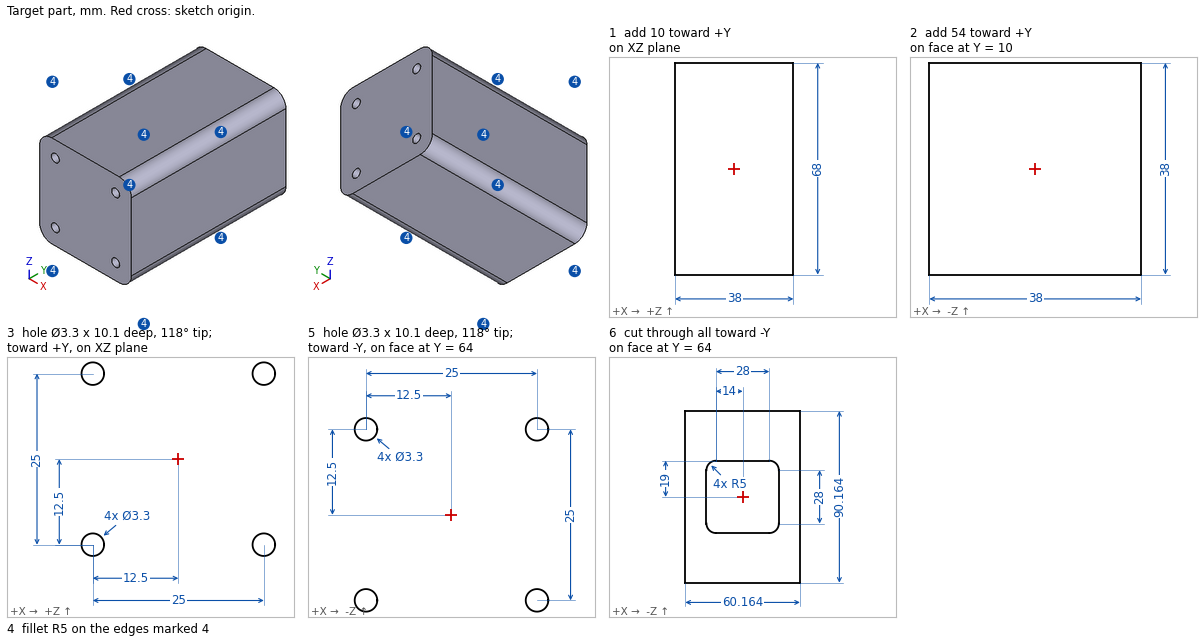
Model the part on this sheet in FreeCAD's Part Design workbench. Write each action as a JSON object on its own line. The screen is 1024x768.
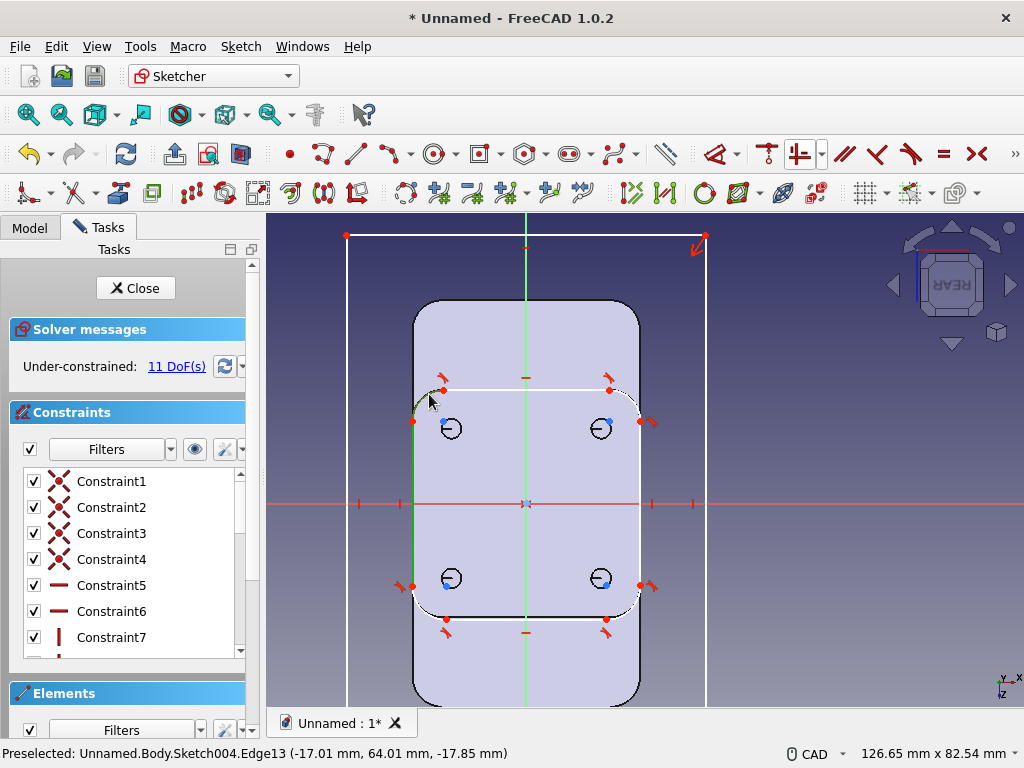
{"action": "left_click", "coordinate": [911, 154]}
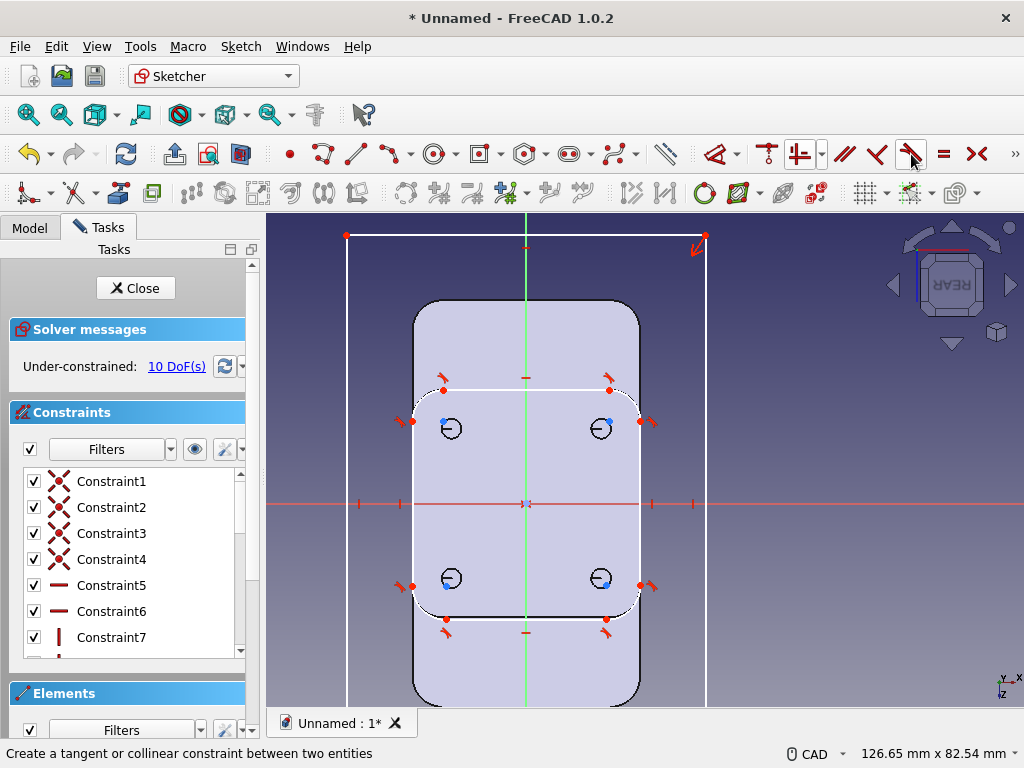
{"action": "left_click", "coordinate": [637, 407]}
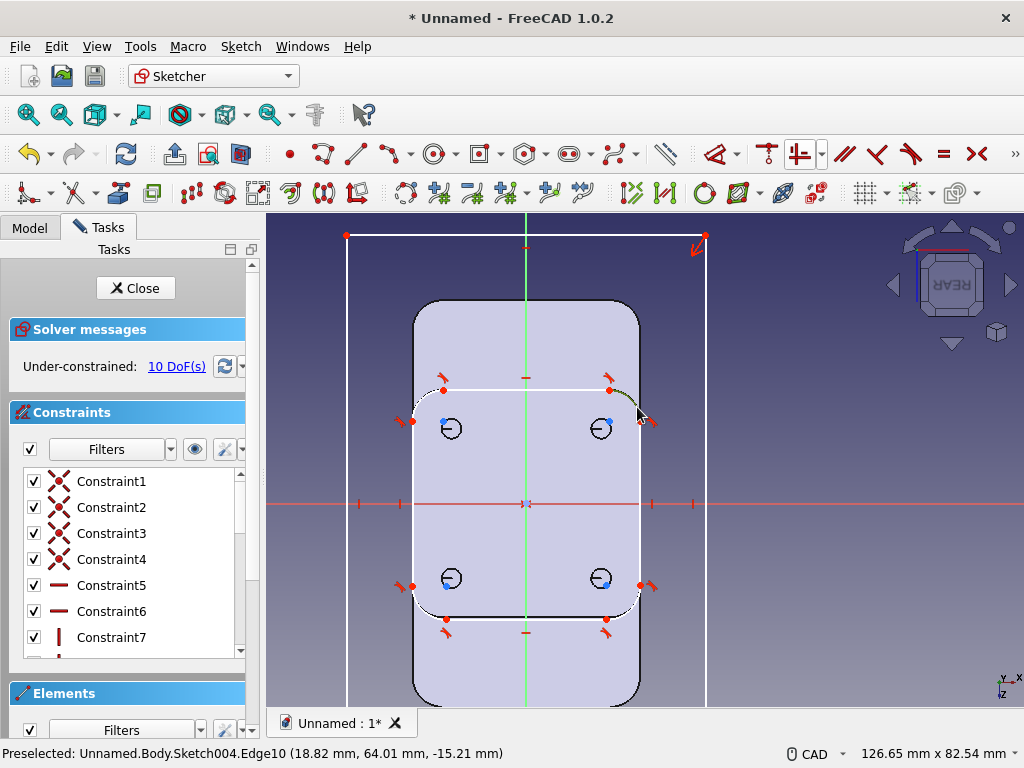
{"action": "left_click", "coordinate": [622, 616]}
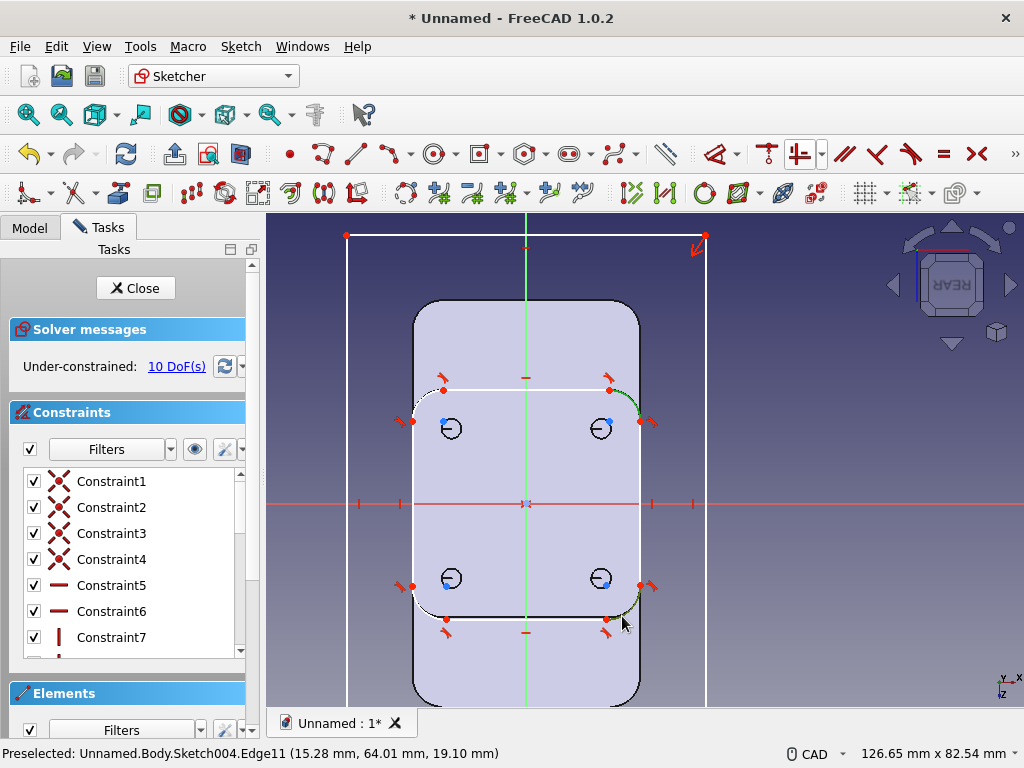
{"action": "left_click", "coordinate": [416, 601]}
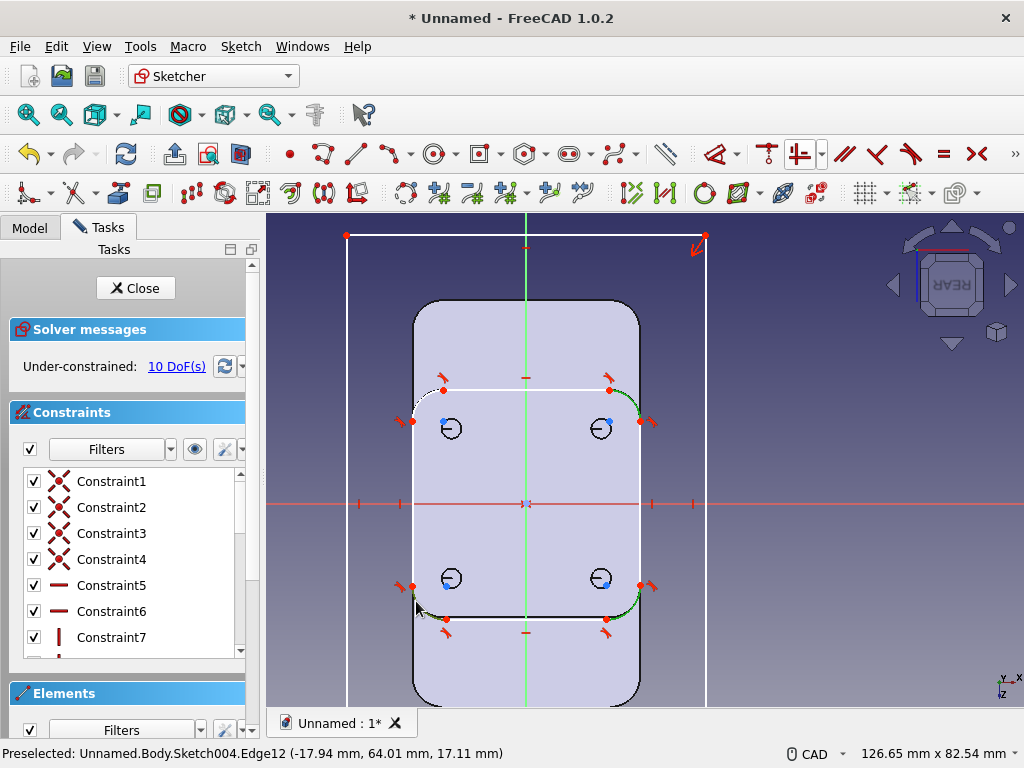
{"action": "left_click", "coordinate": [429, 394]}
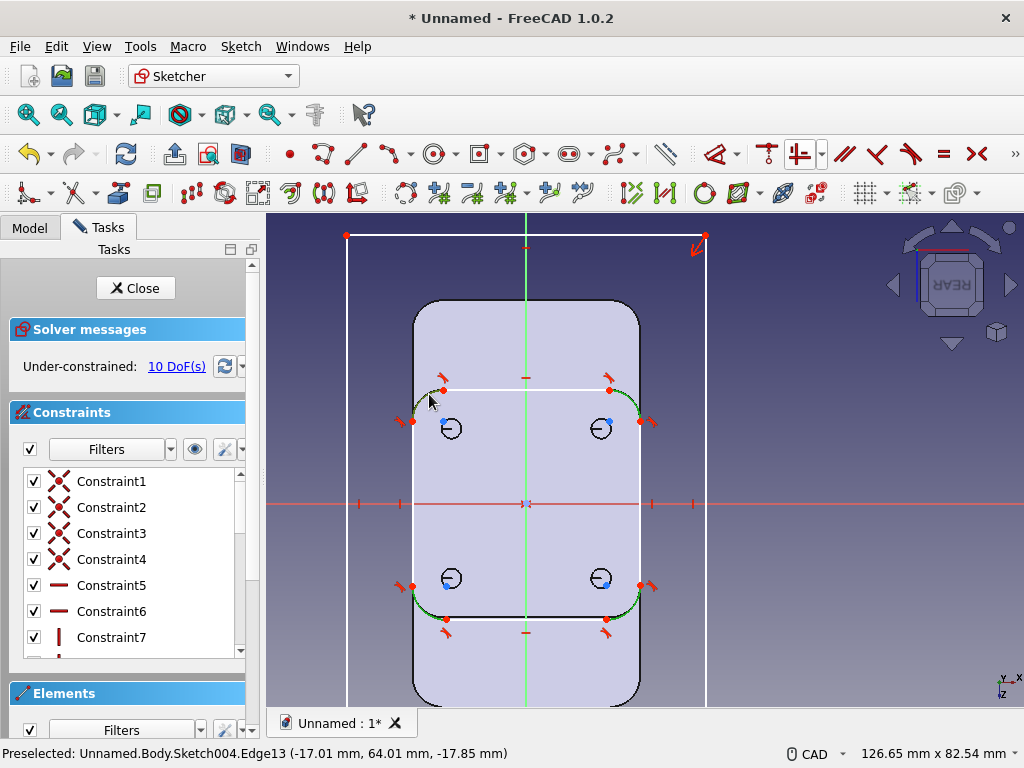
{"action": "left_click", "coordinate": [944, 154]}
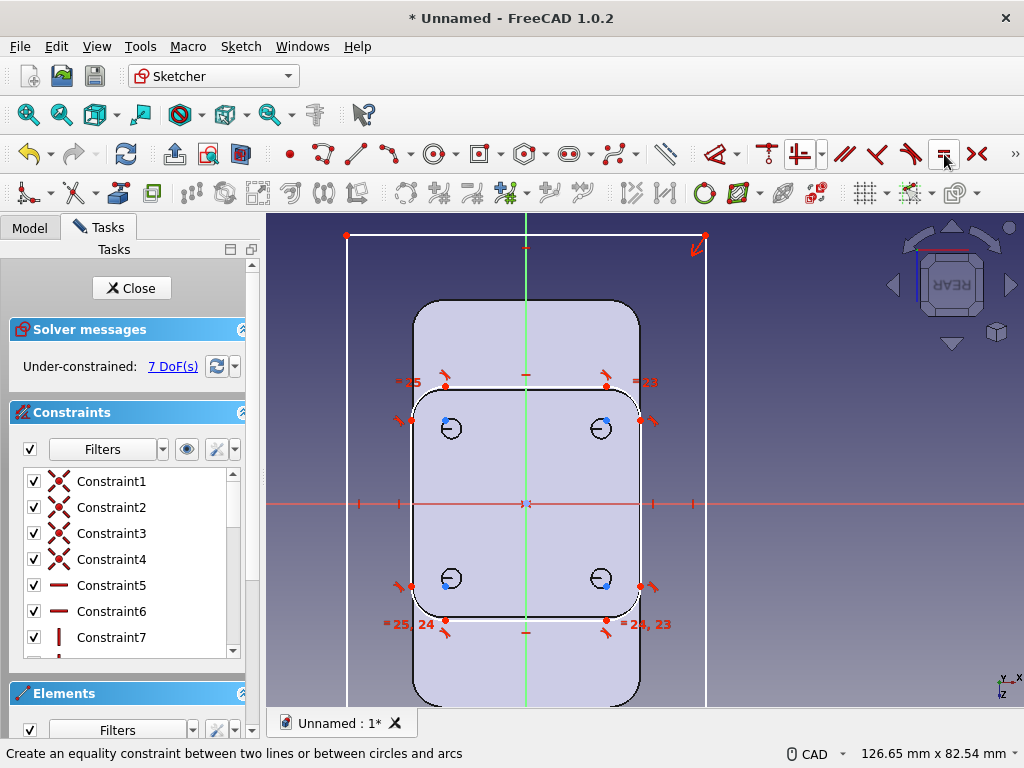
{"action": "left_click", "coordinate": [714, 154]}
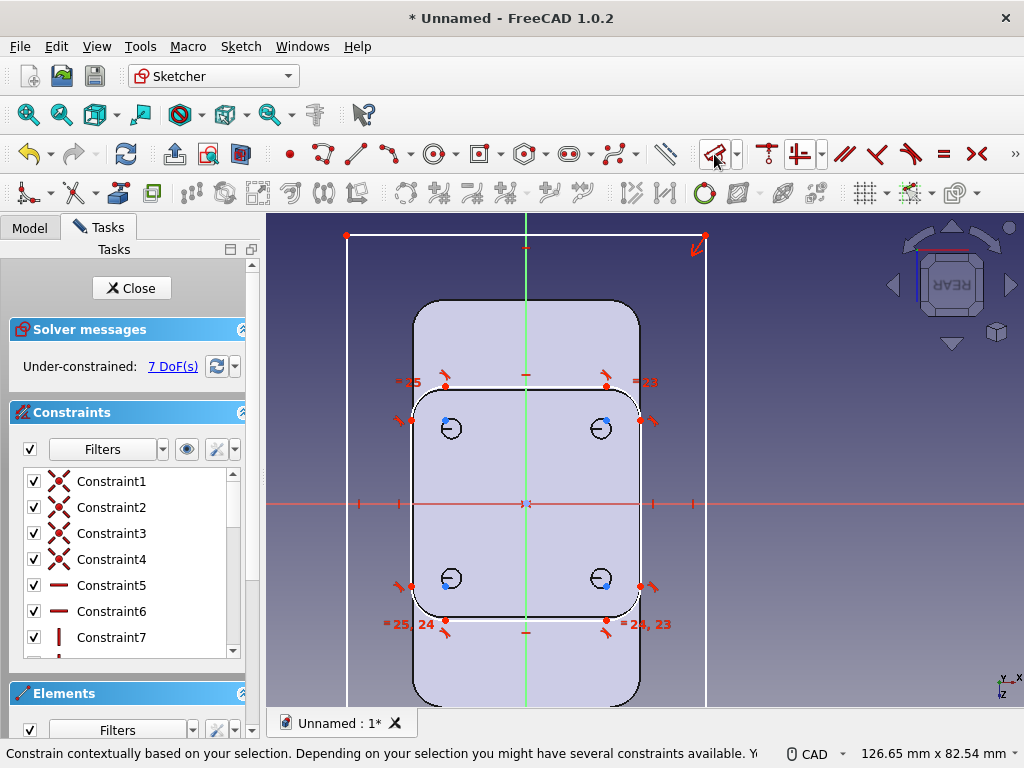
{"action": "scroll", "coordinate": [637, 405], "scroll_direction": "up", "scroll_amount": 2}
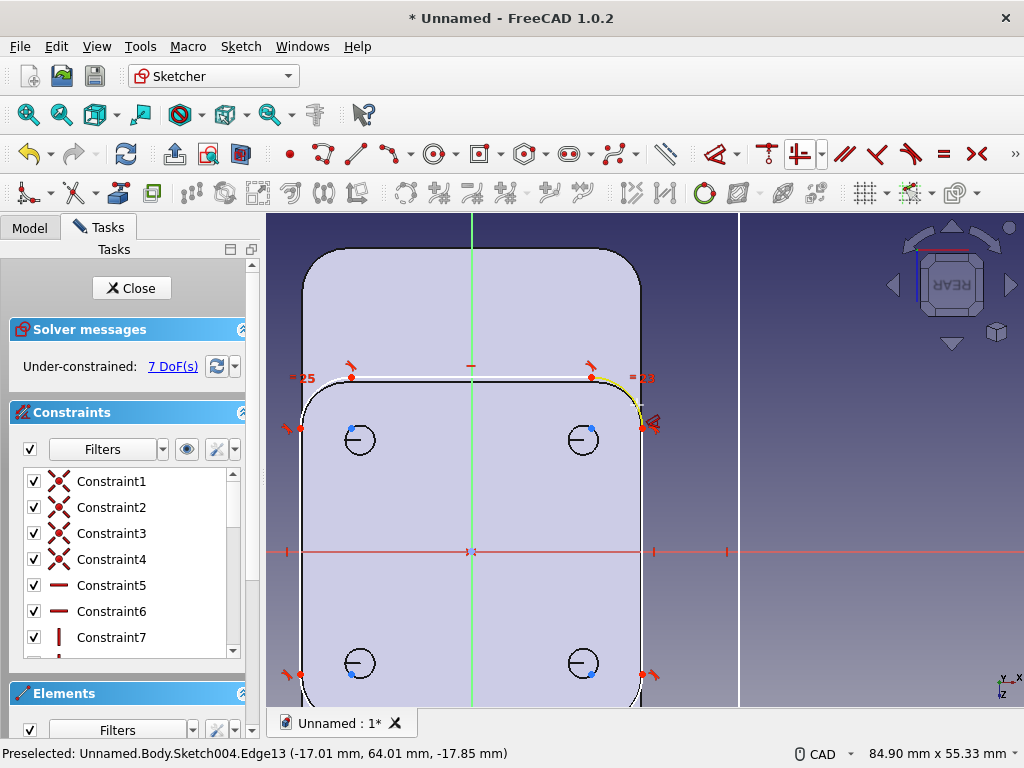
{"action": "left_click", "coordinate": [637, 405]}
{"action": "left_click", "coordinate": [665, 390]}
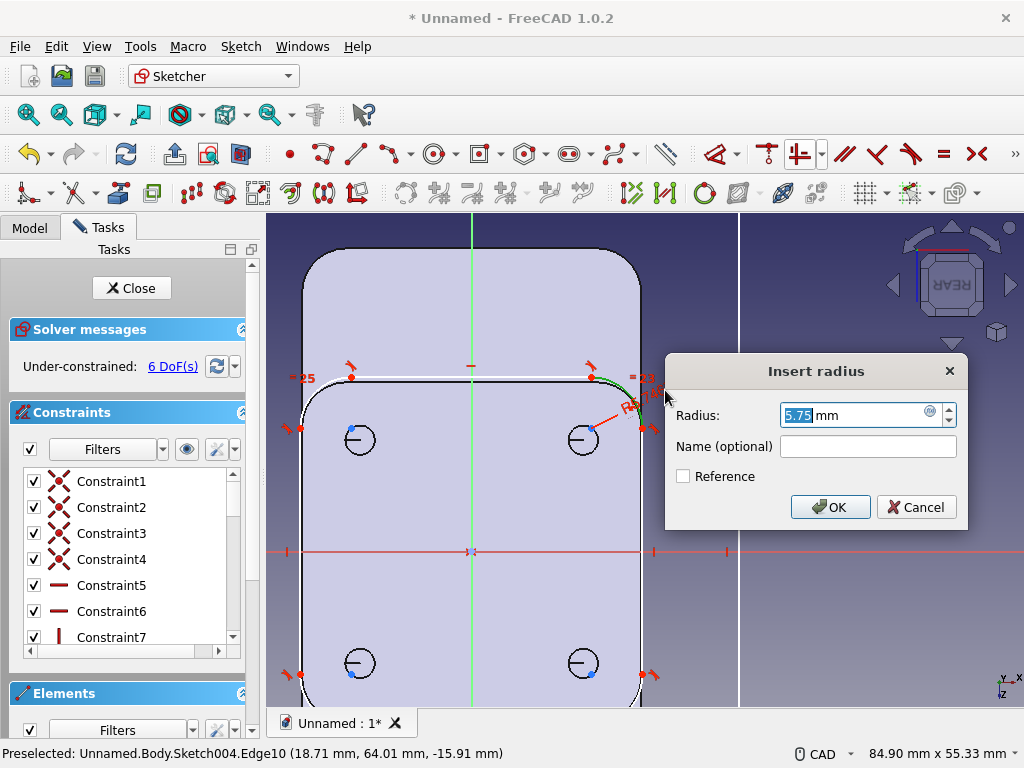
{"action": "type", "text": "5"}
{"action": "key", "text": "Return"}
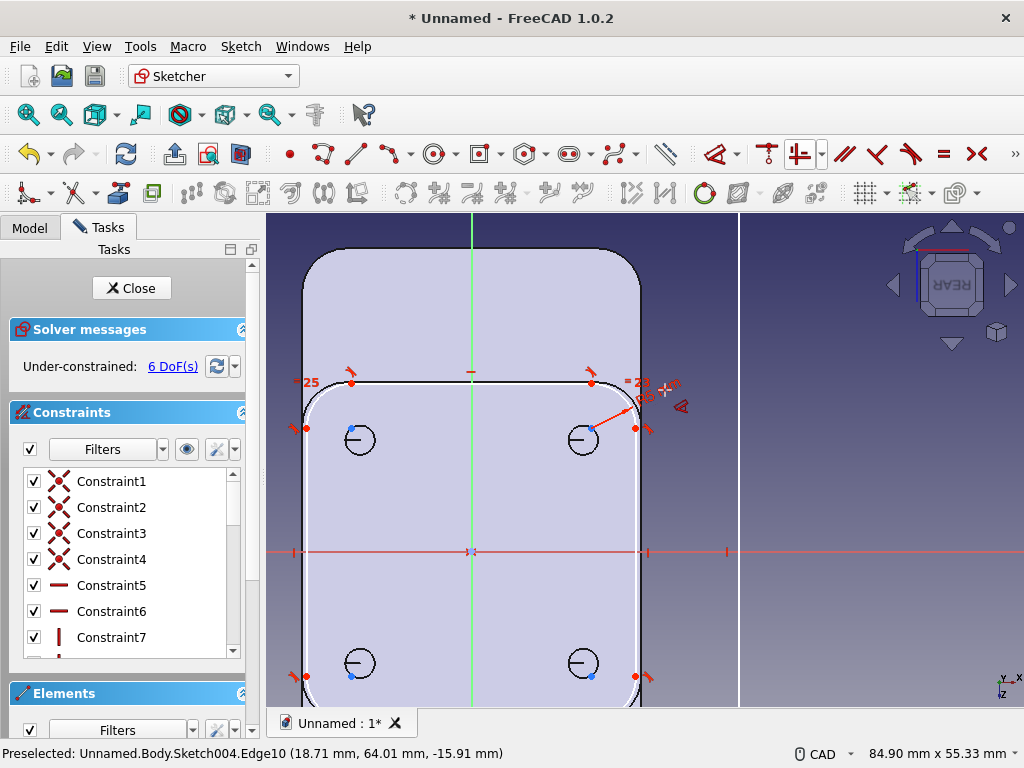
{"action": "left_click", "coordinate": [423, 384]}
{"action": "left_click", "coordinate": [416, 350]}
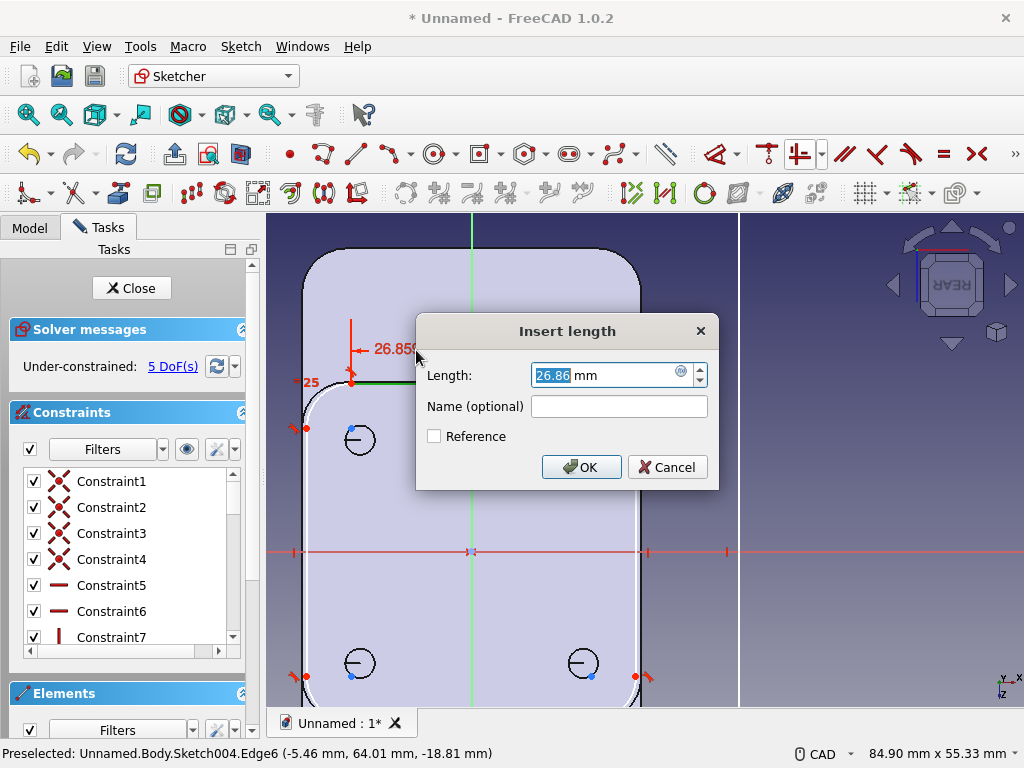
{"action": "type", "text": "28"}
{"action": "key", "text": "Return"}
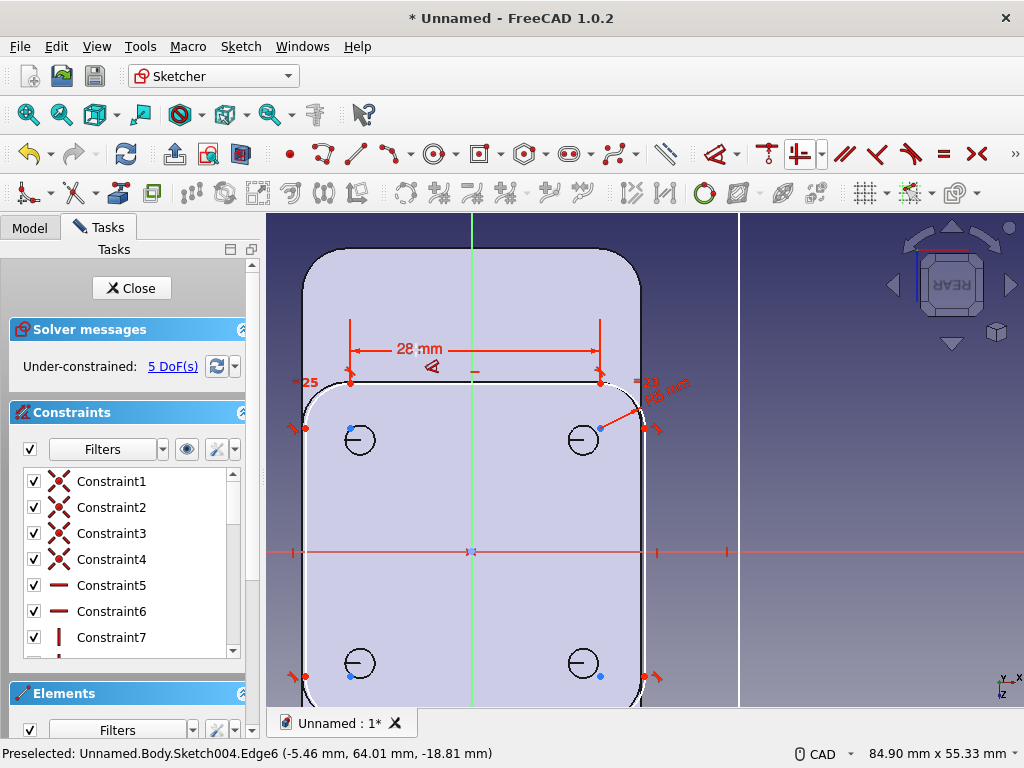
{"action": "left_click", "coordinate": [645, 503]}
{"action": "left_click", "coordinate": [679, 495]}